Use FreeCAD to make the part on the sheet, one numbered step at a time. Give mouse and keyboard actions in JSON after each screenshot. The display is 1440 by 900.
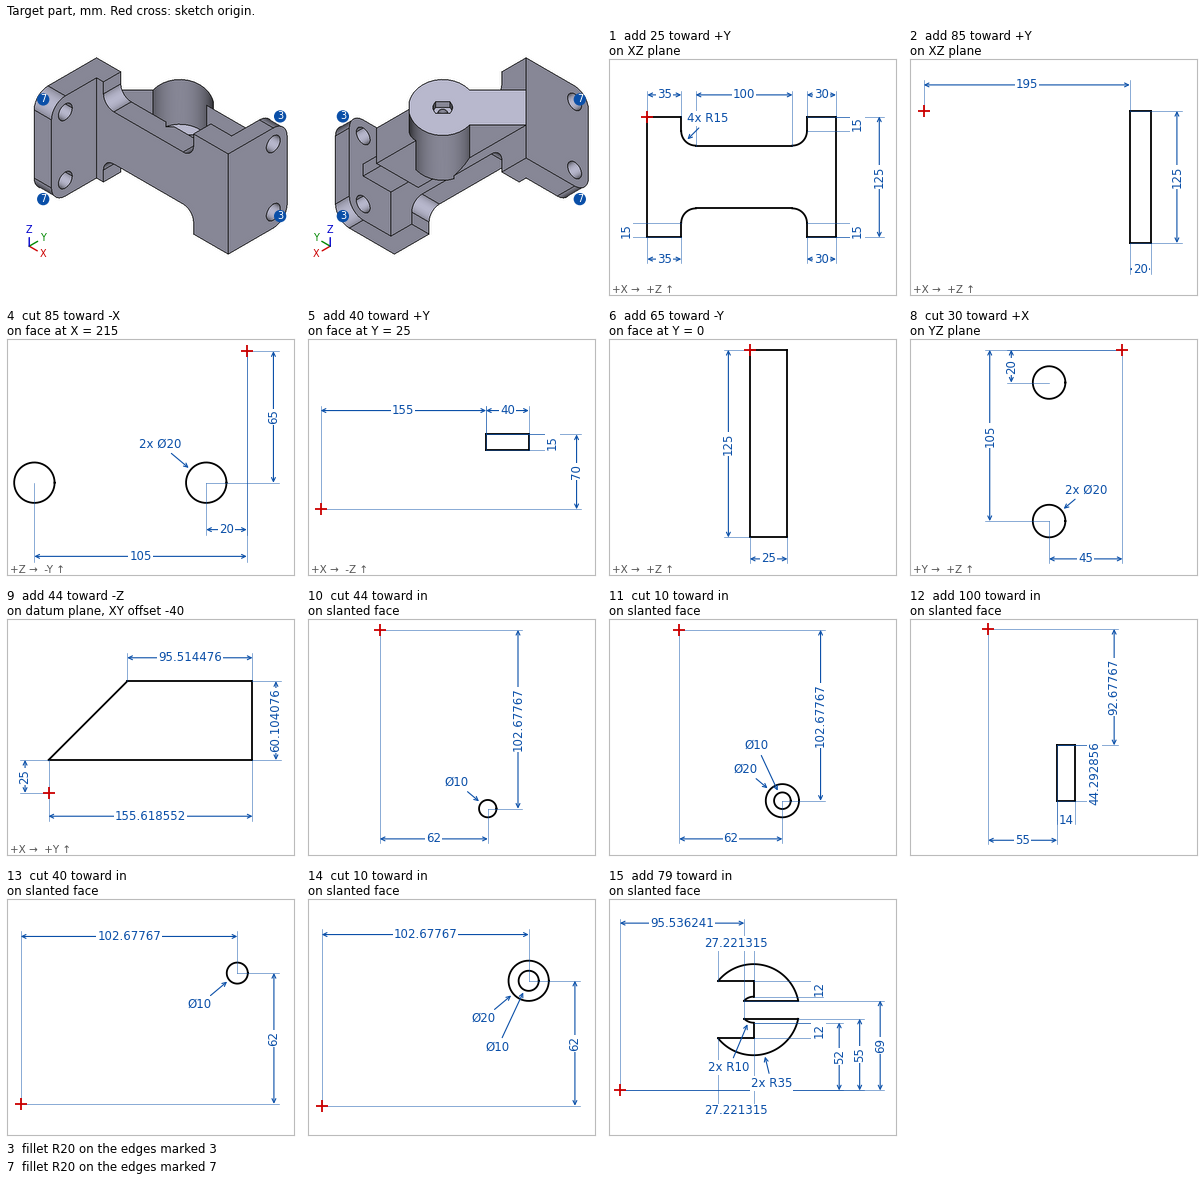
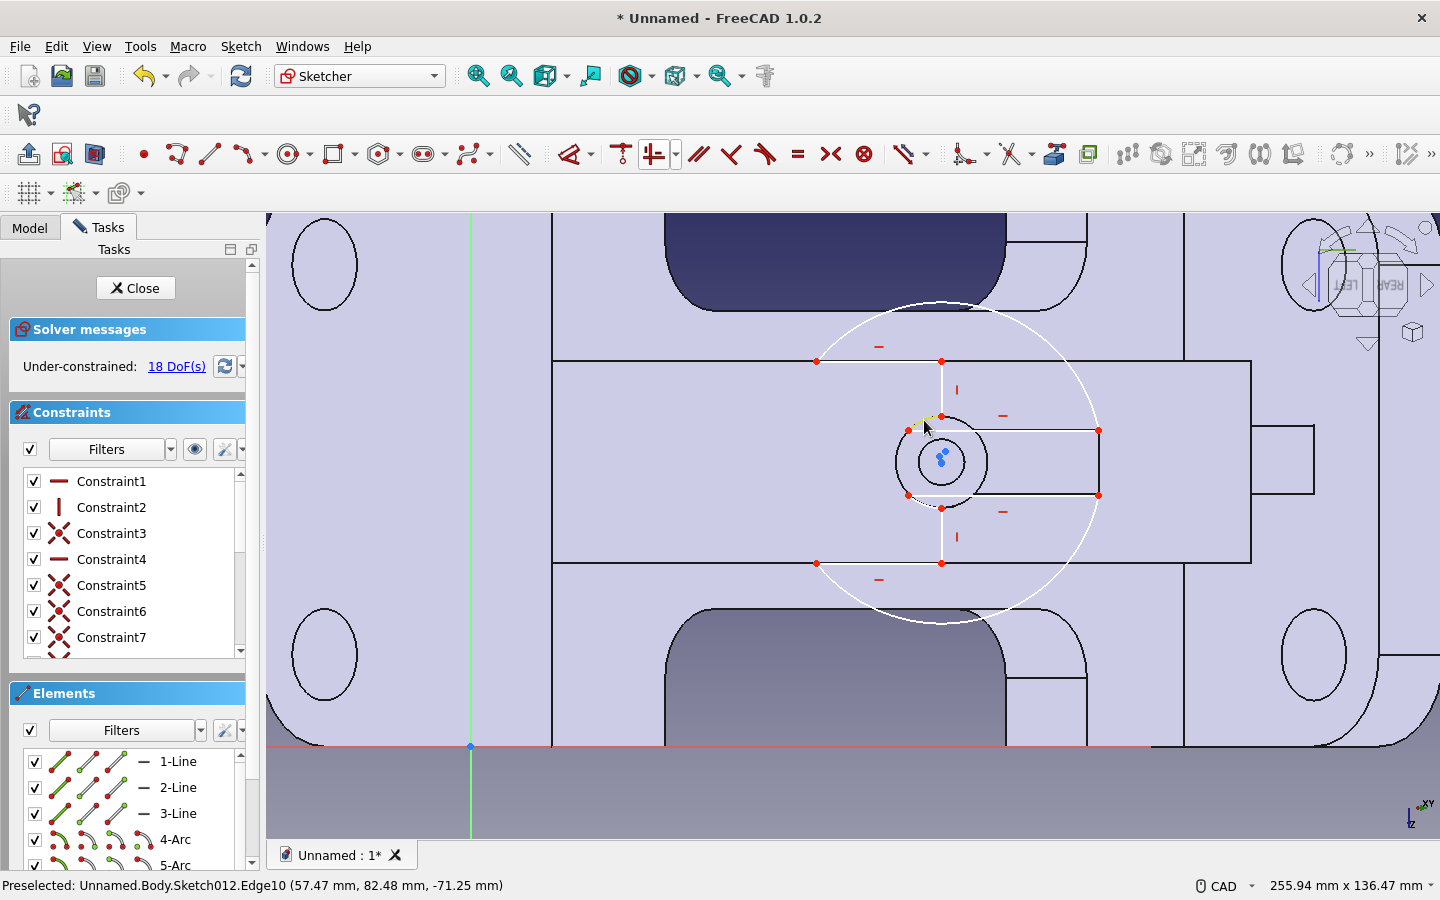
{"action": "scroll", "coordinate": [918, 502], "scroll_direction": "up", "scroll_amount": 5}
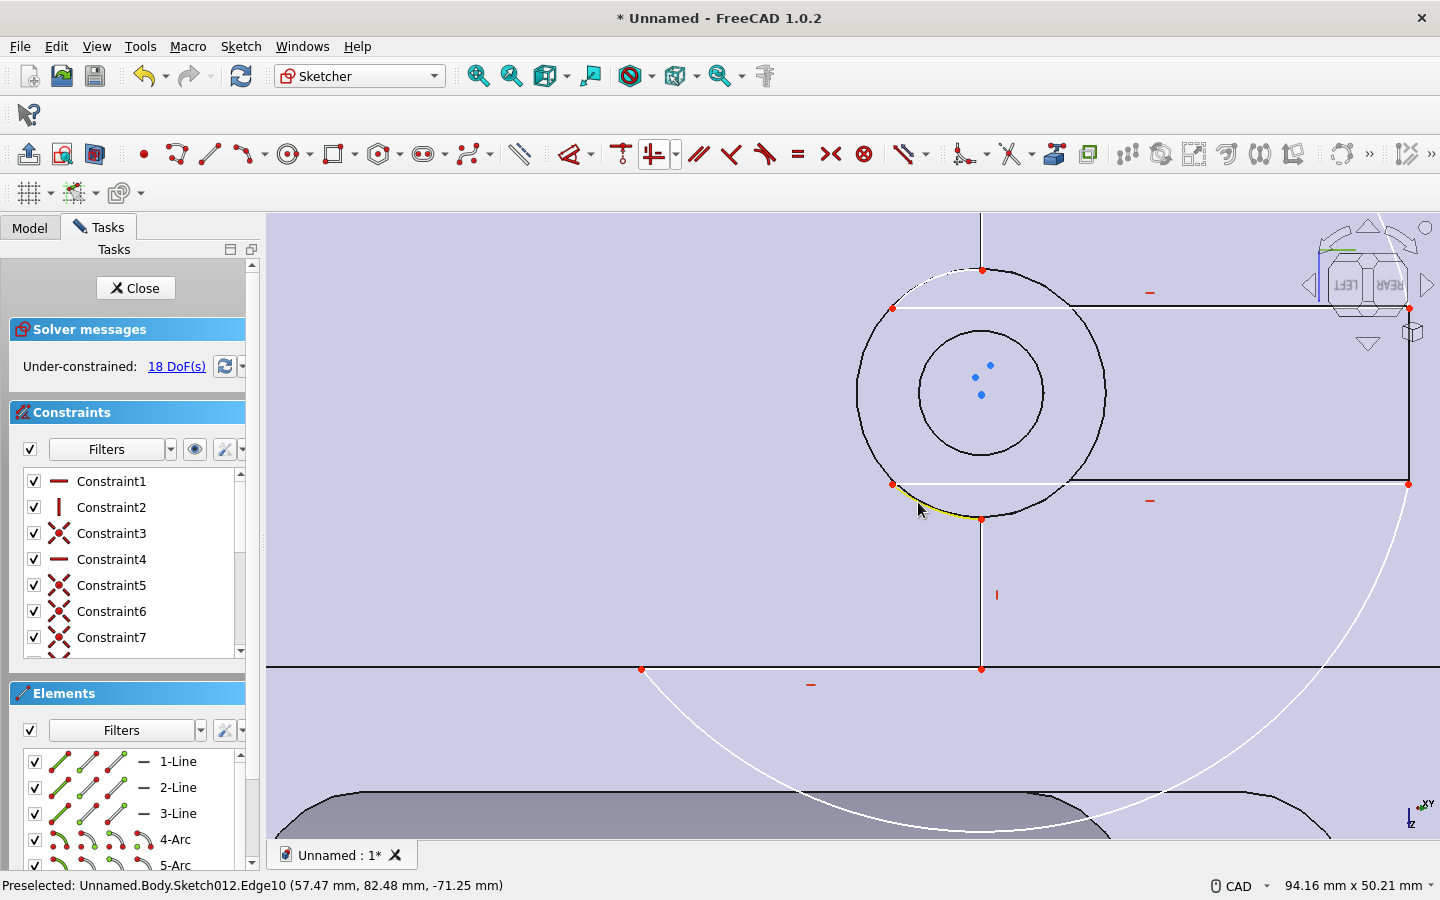
{"action": "left_click", "coordinate": [916, 501]}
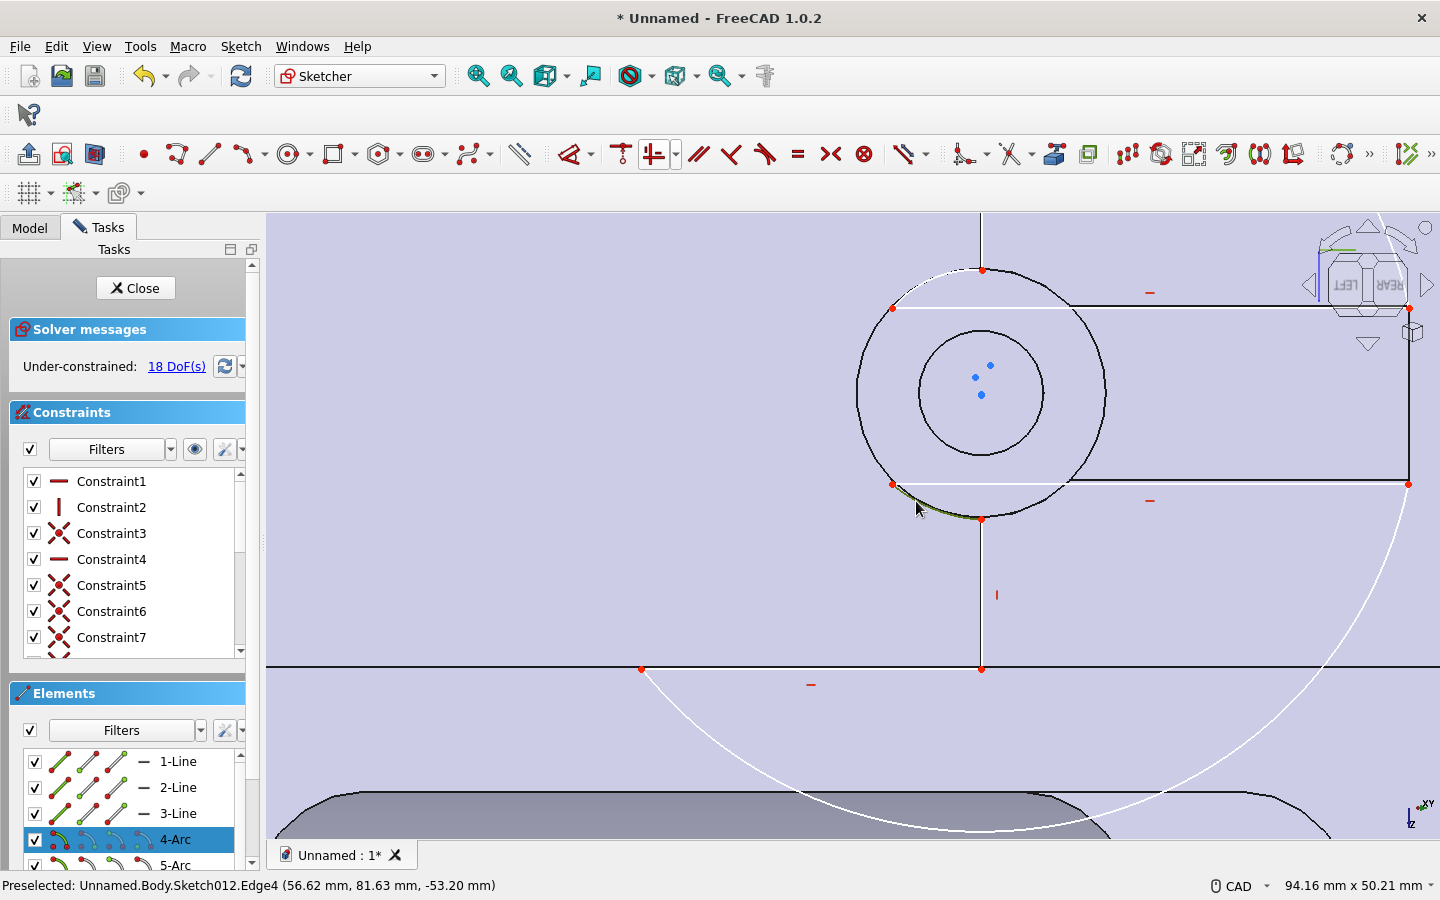
{"action": "left_click", "coordinate": [1259, 733]}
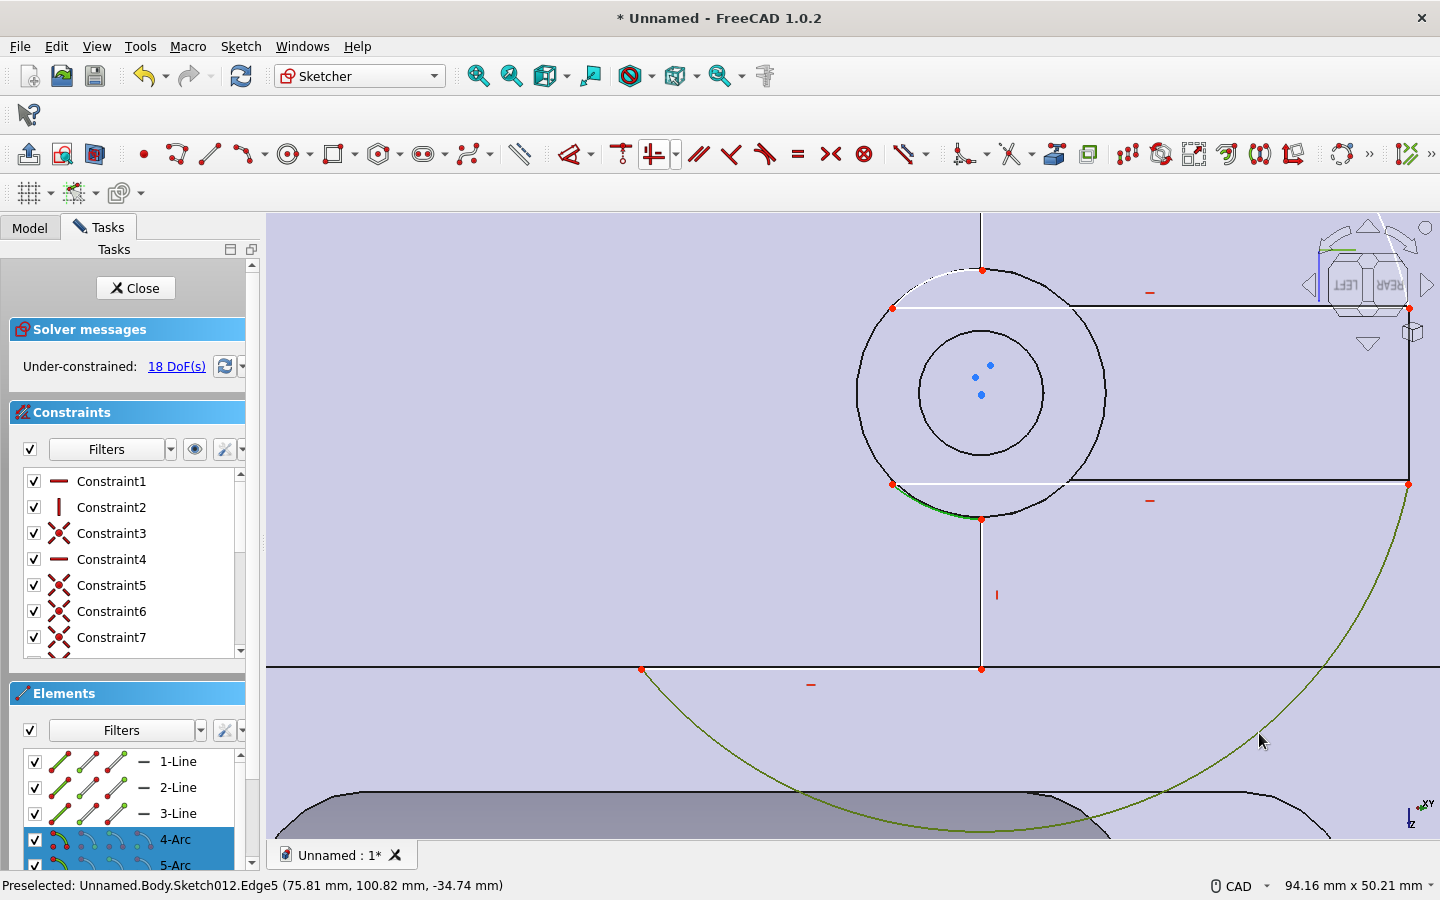
{"action": "left_click", "coordinate": [621, 154]}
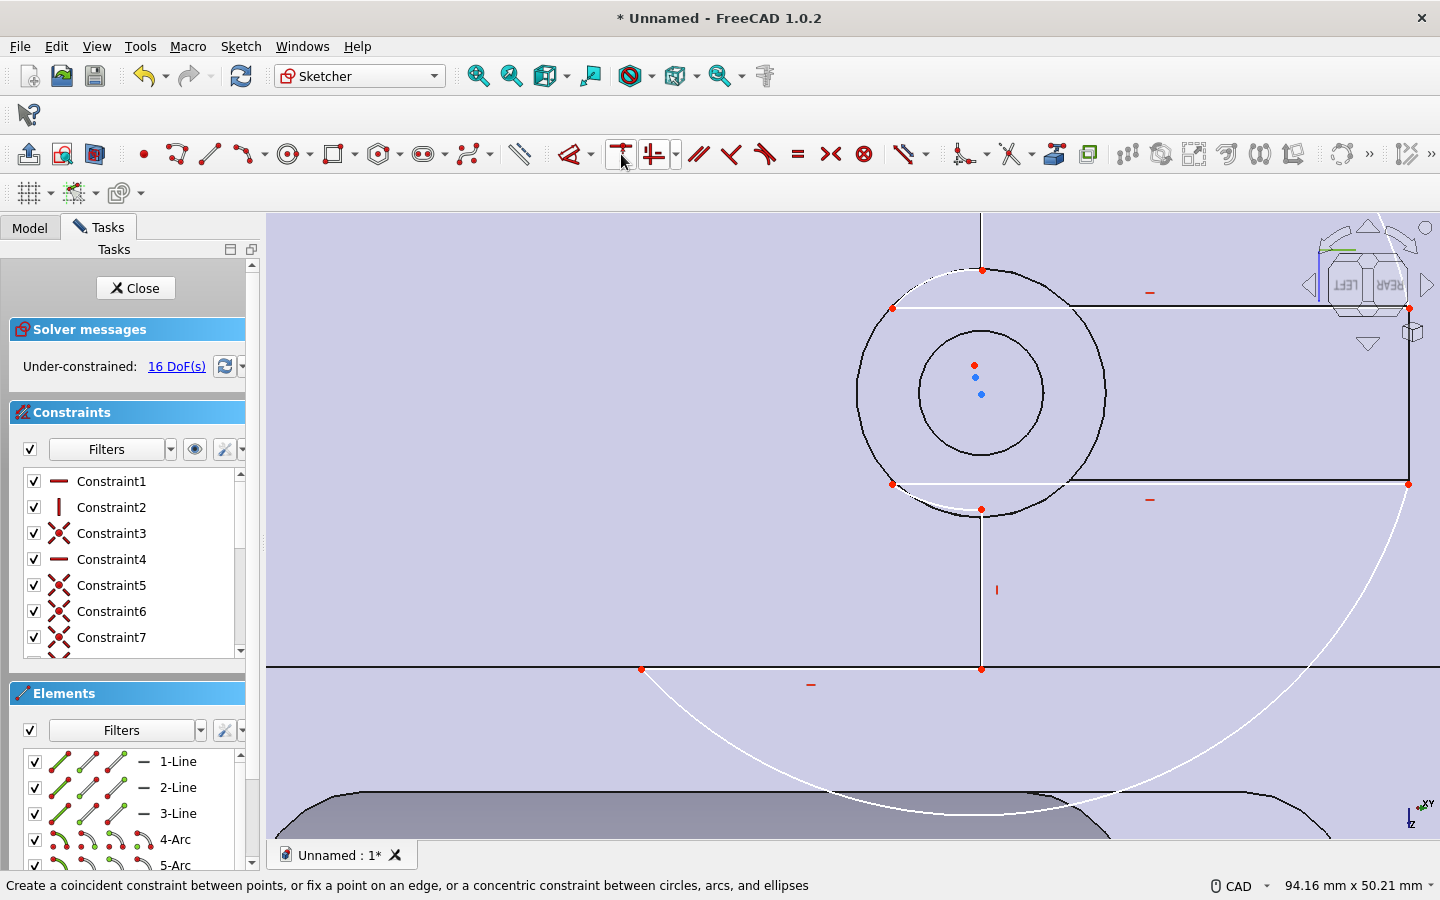
{"action": "left_click", "coordinate": [917, 498]}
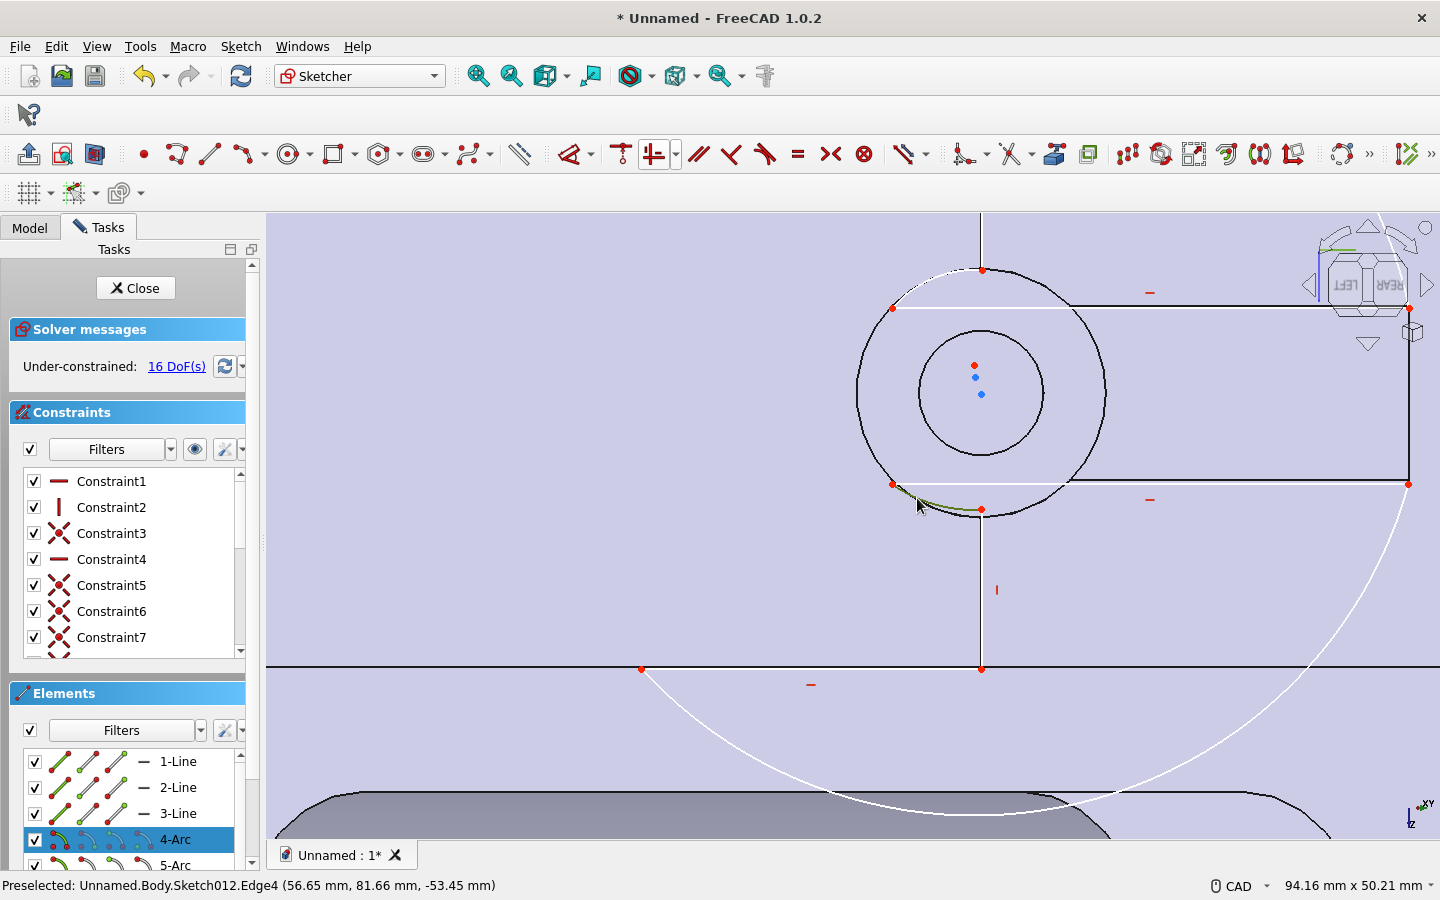
{"action": "scroll", "coordinate": [918, 502], "scroll_direction": "down", "scroll_amount": 5}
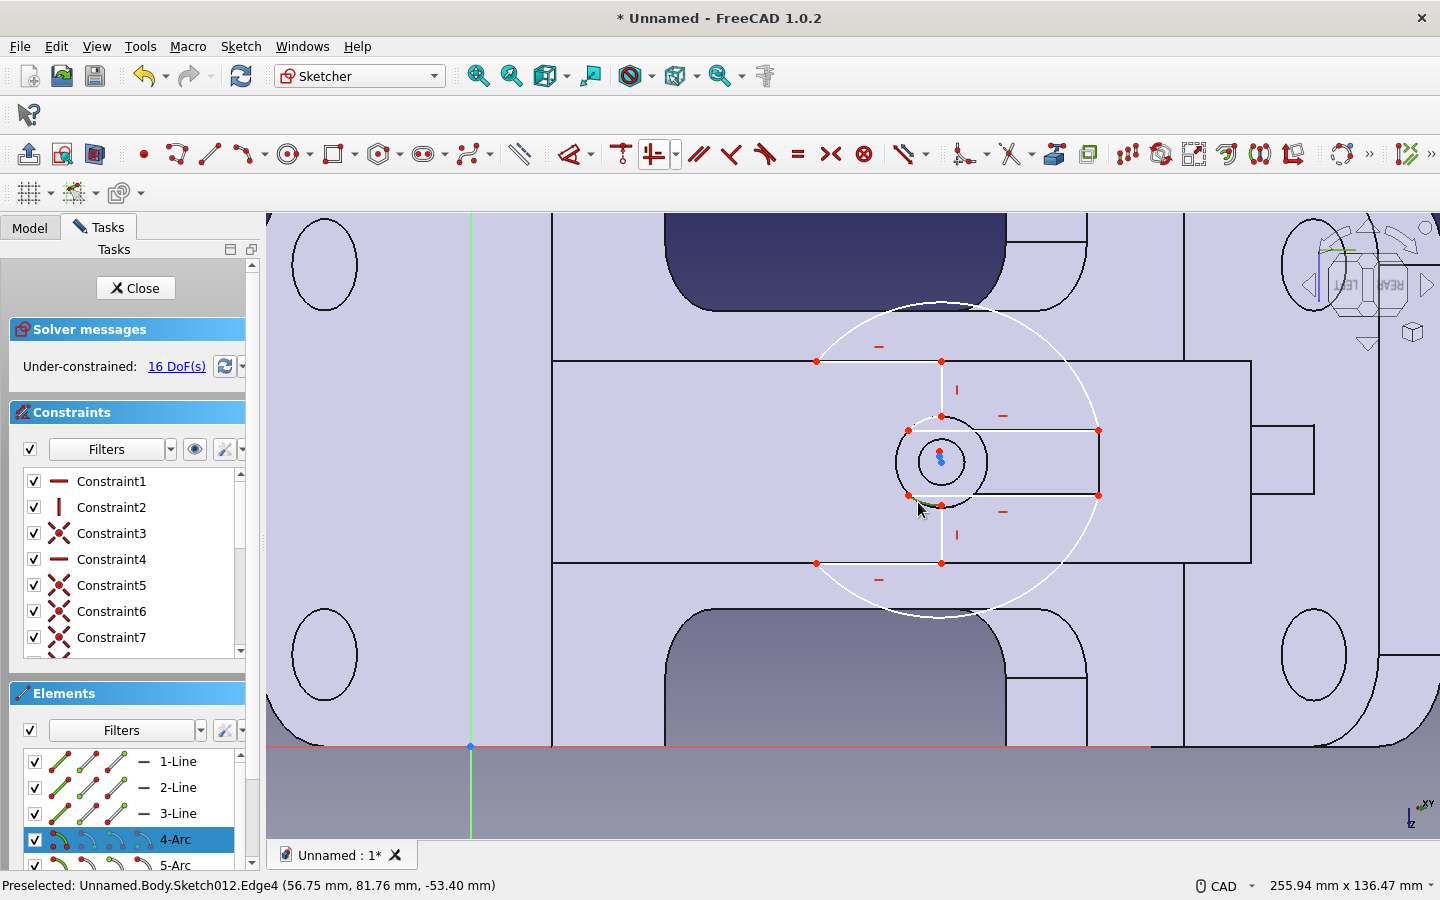
{"action": "left_click", "coordinate": [1044, 339]}